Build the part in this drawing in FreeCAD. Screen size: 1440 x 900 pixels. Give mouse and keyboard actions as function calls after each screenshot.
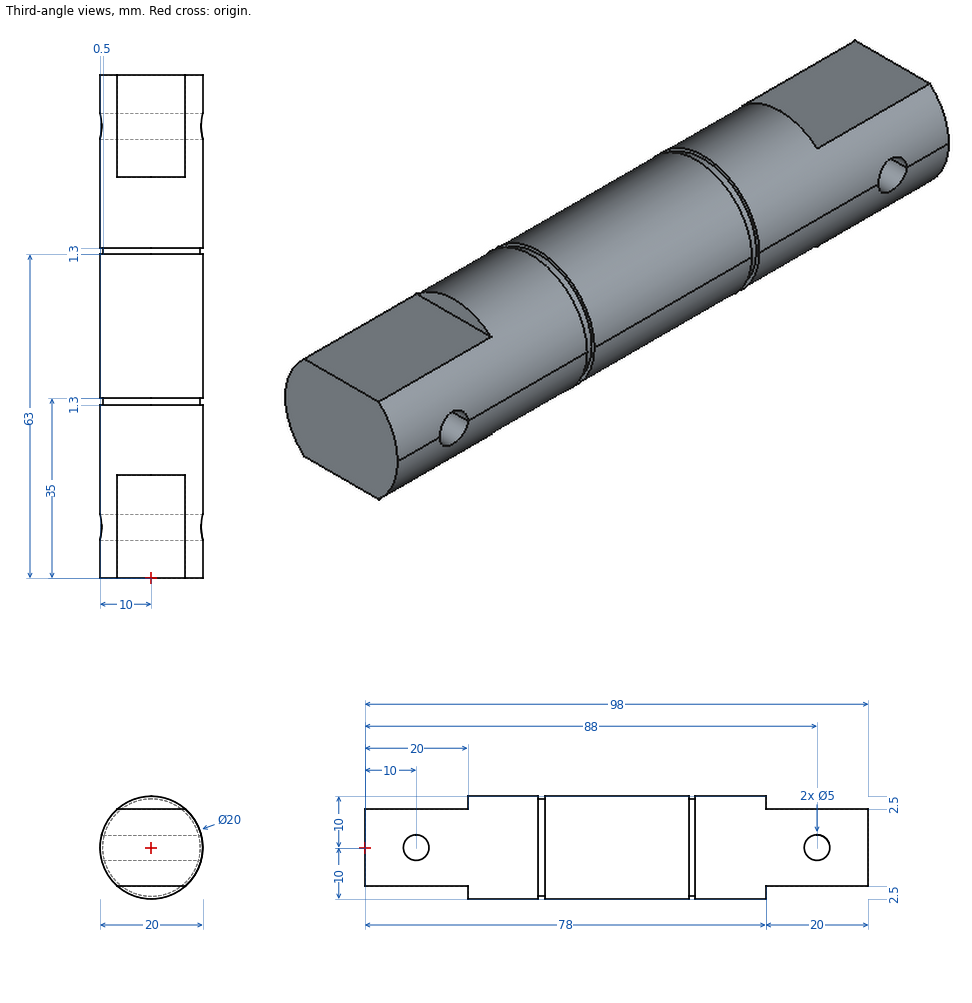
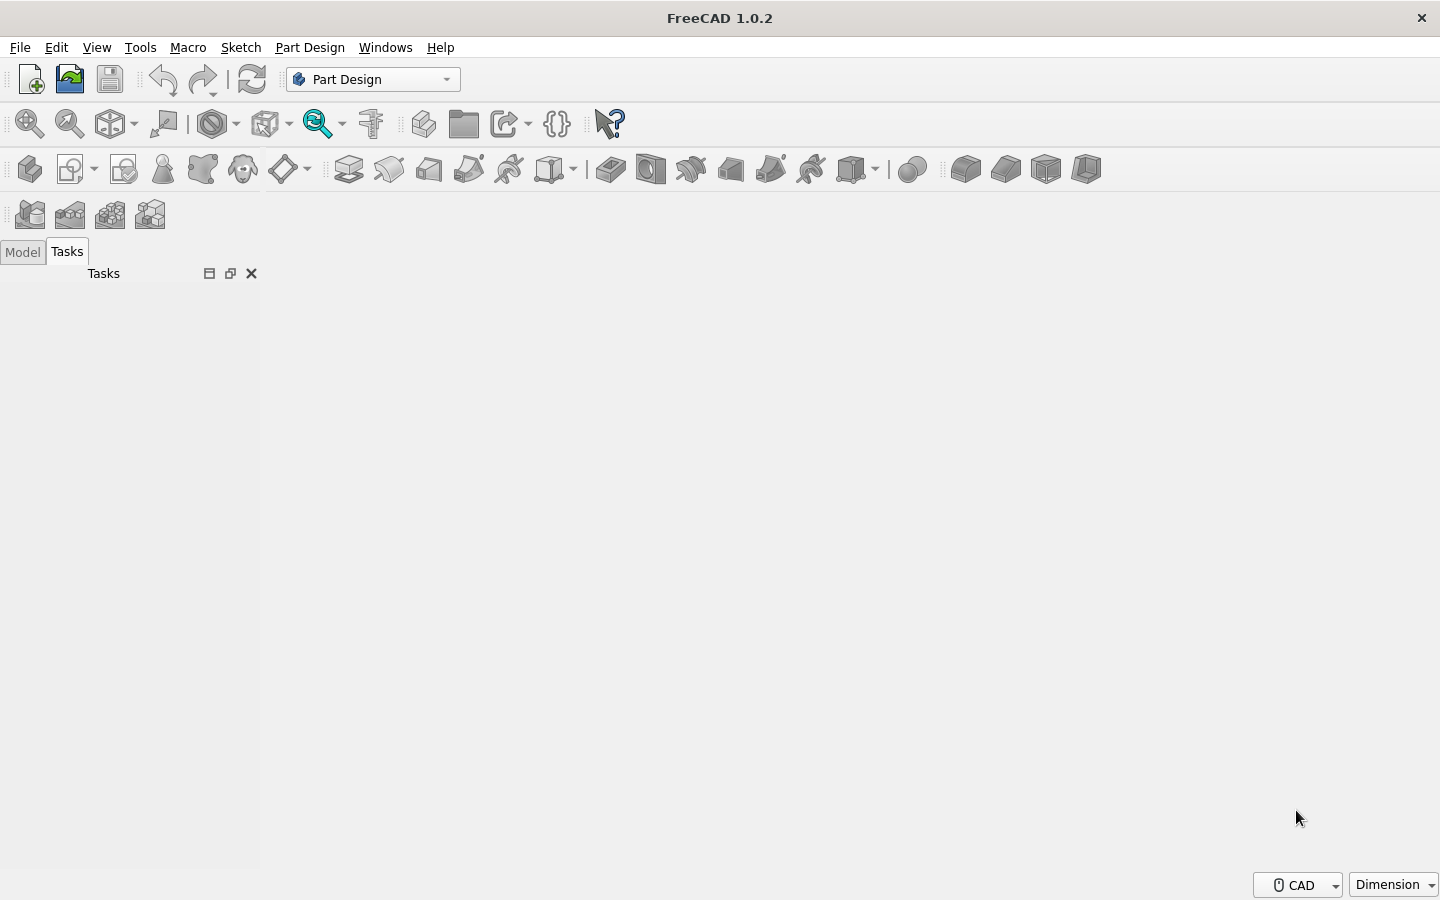
click(30, 80)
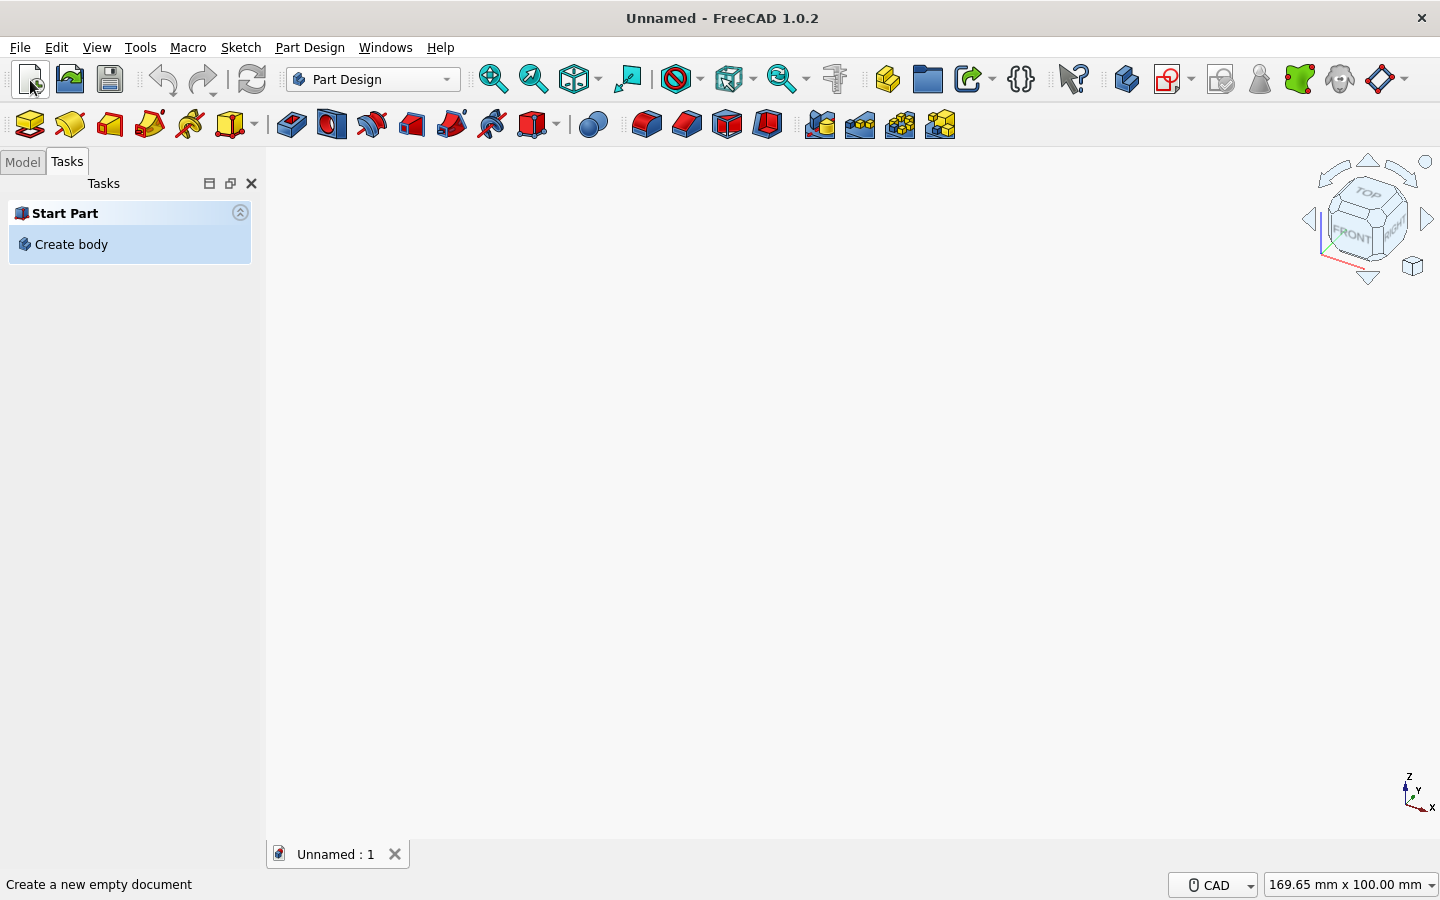
click(1168, 80)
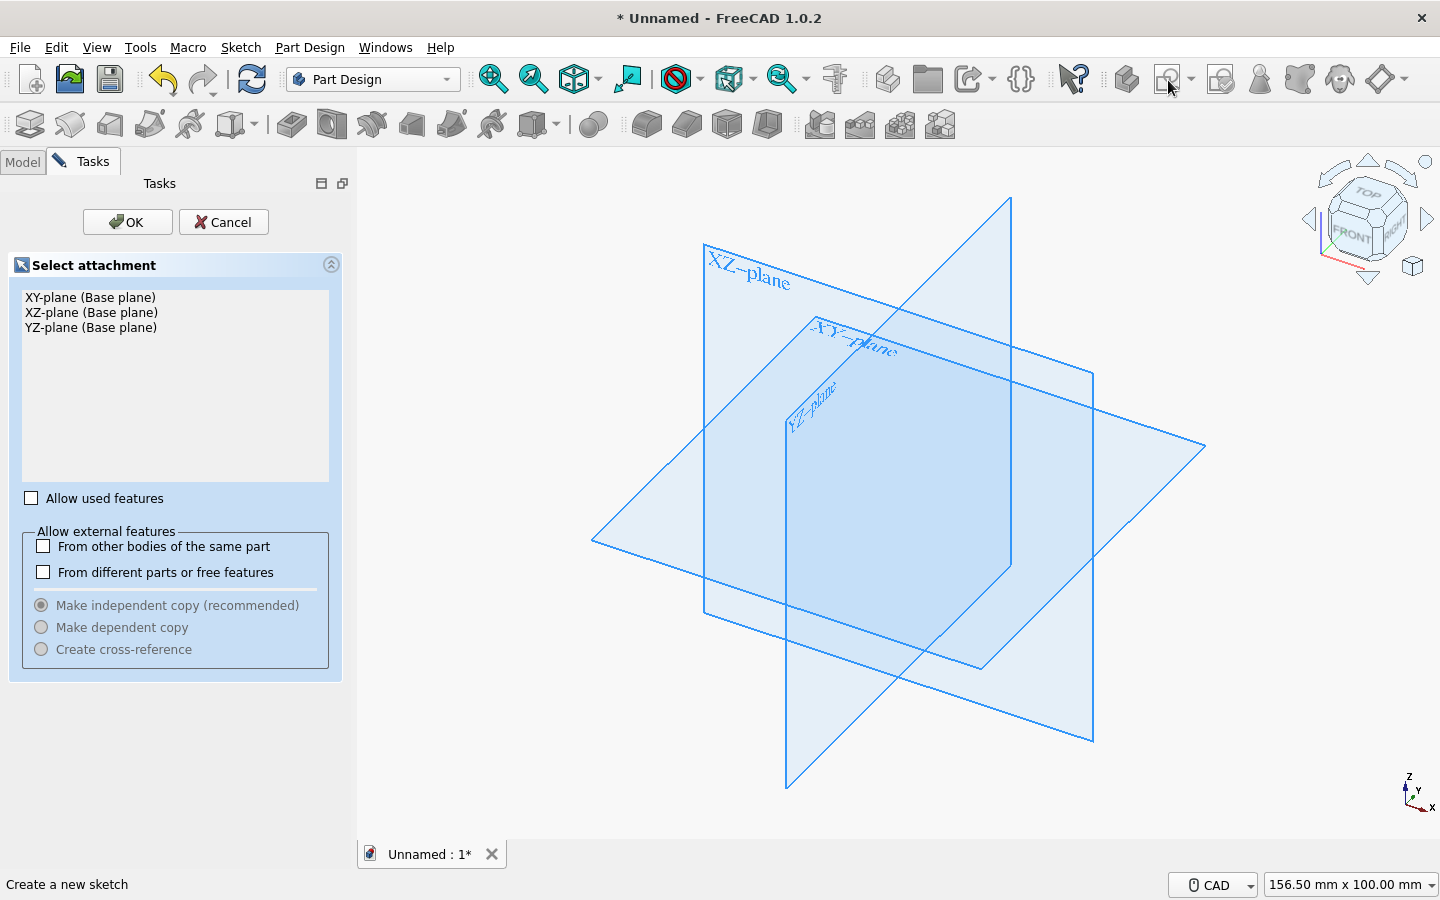
click(82, 312)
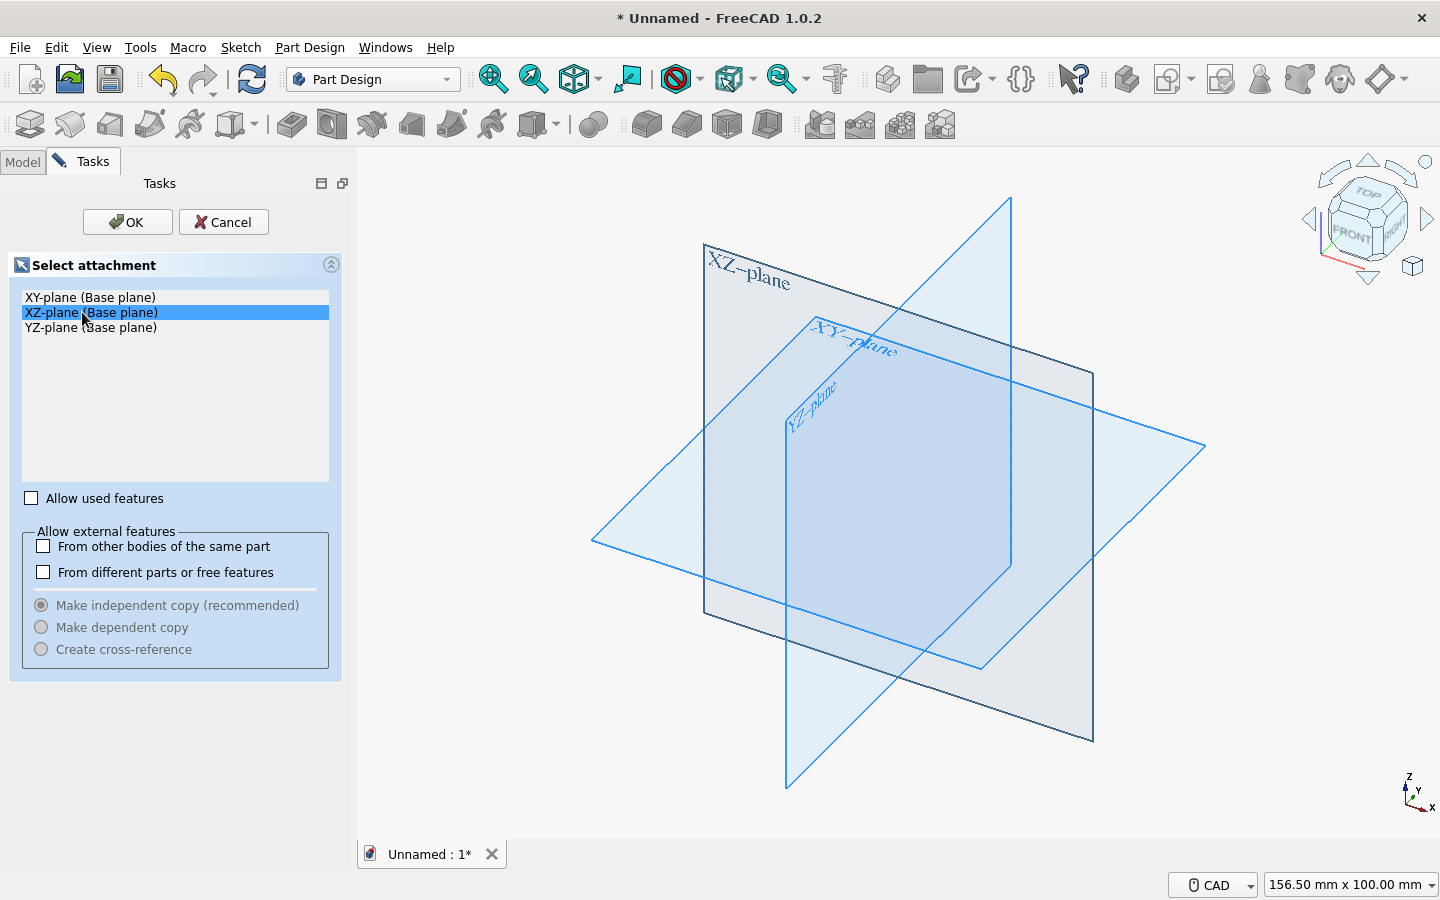
click(128, 222)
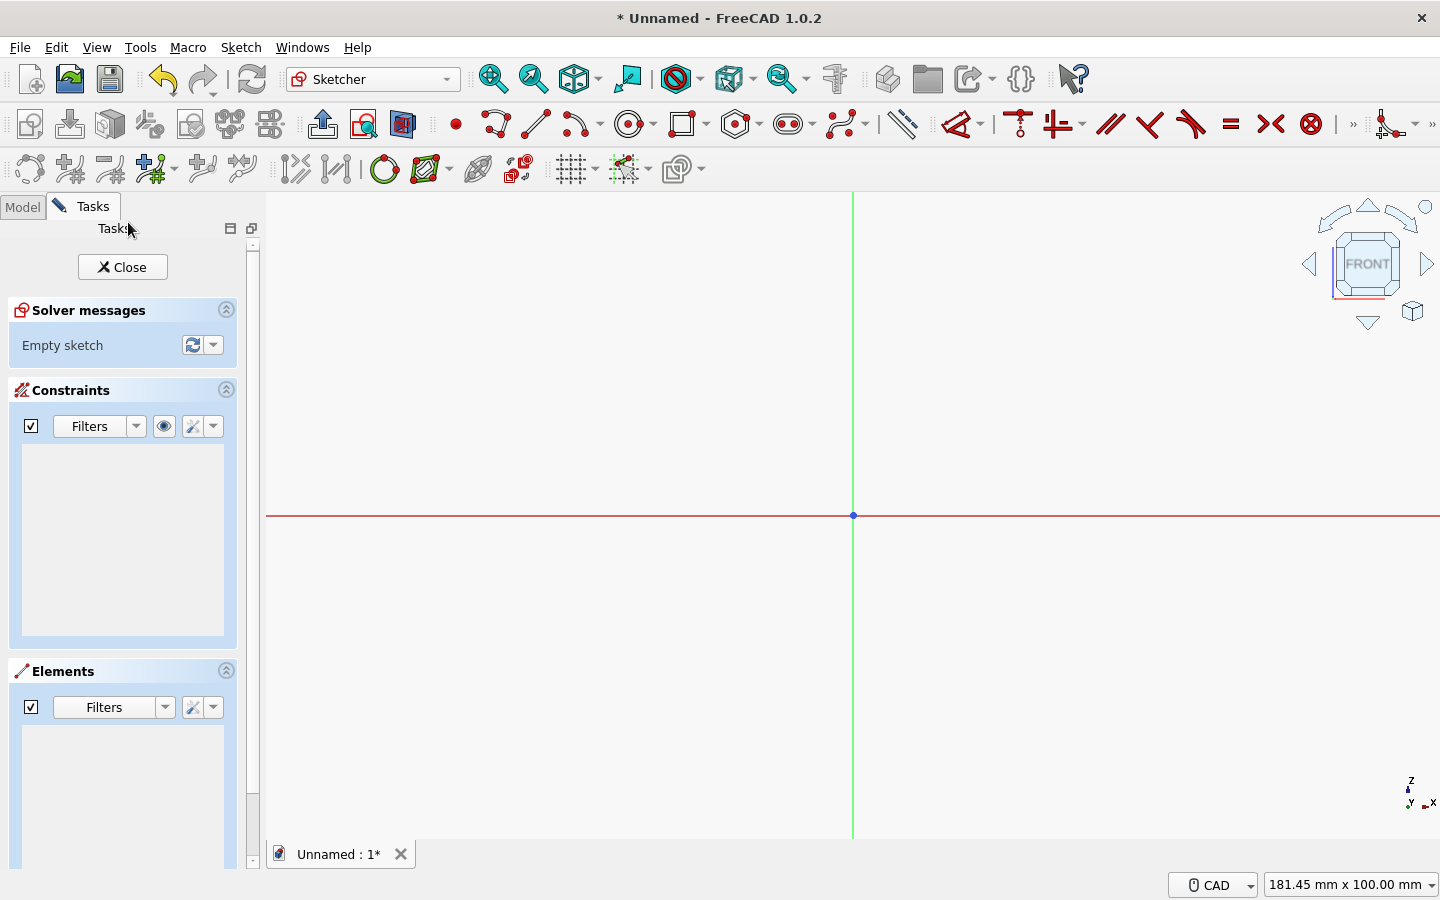
scroll(883, 516, up, 6)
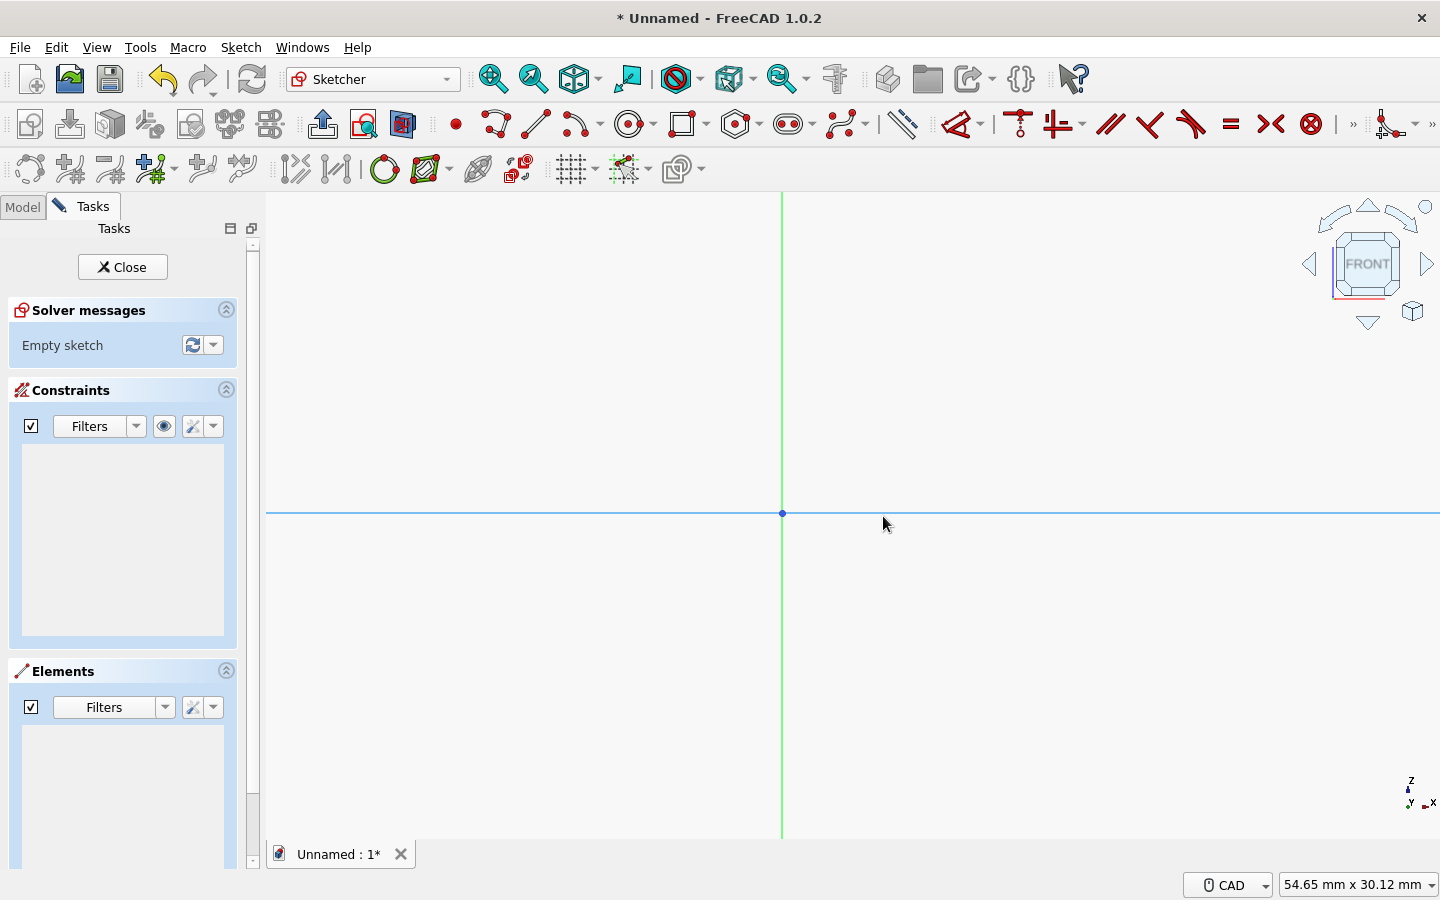
click(630, 124)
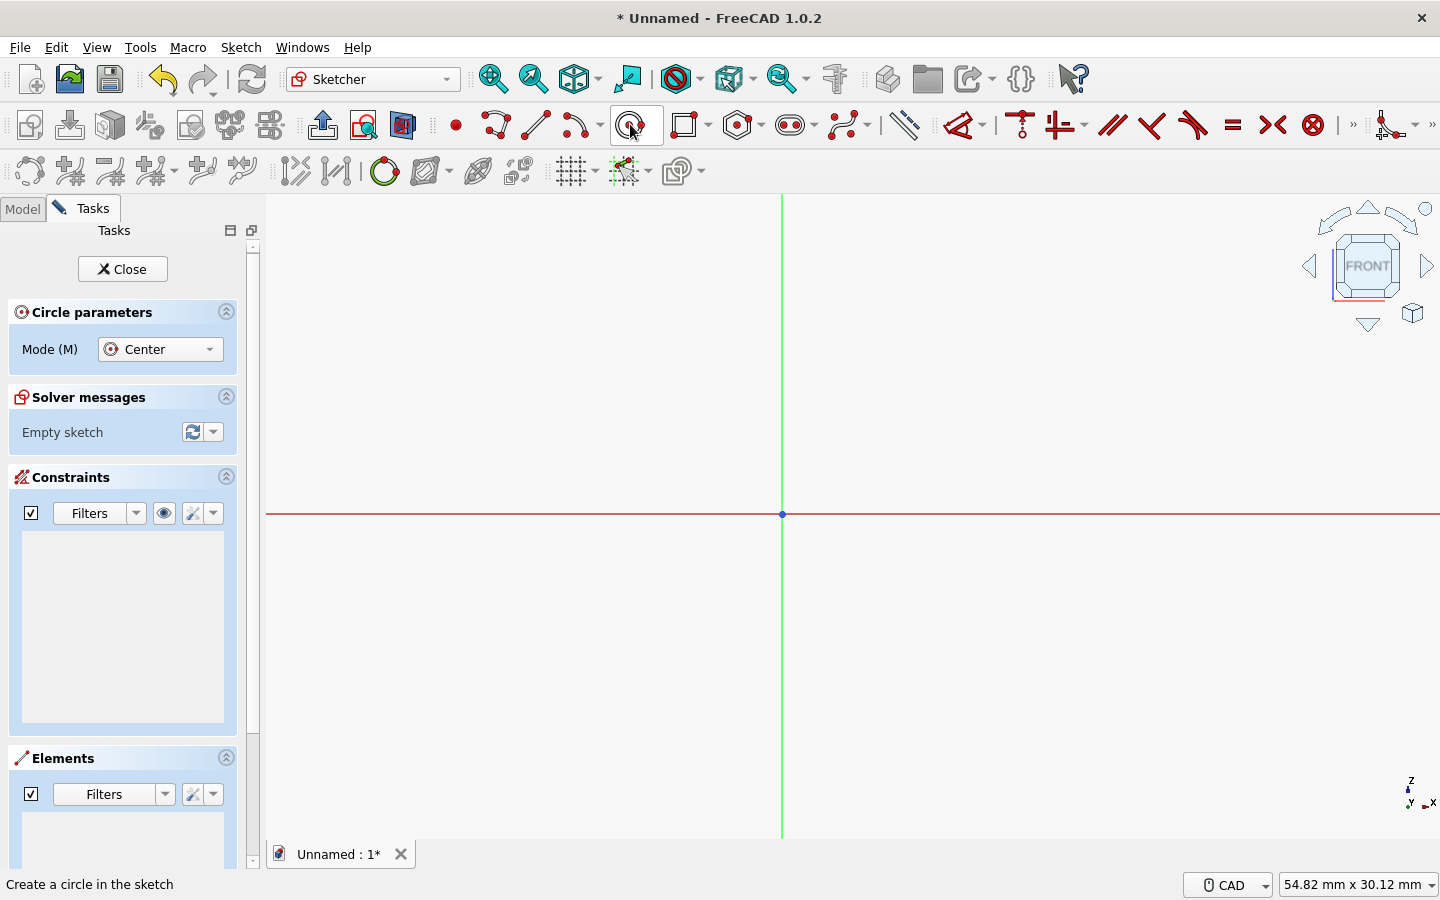
click(782, 514)
move(934, 363)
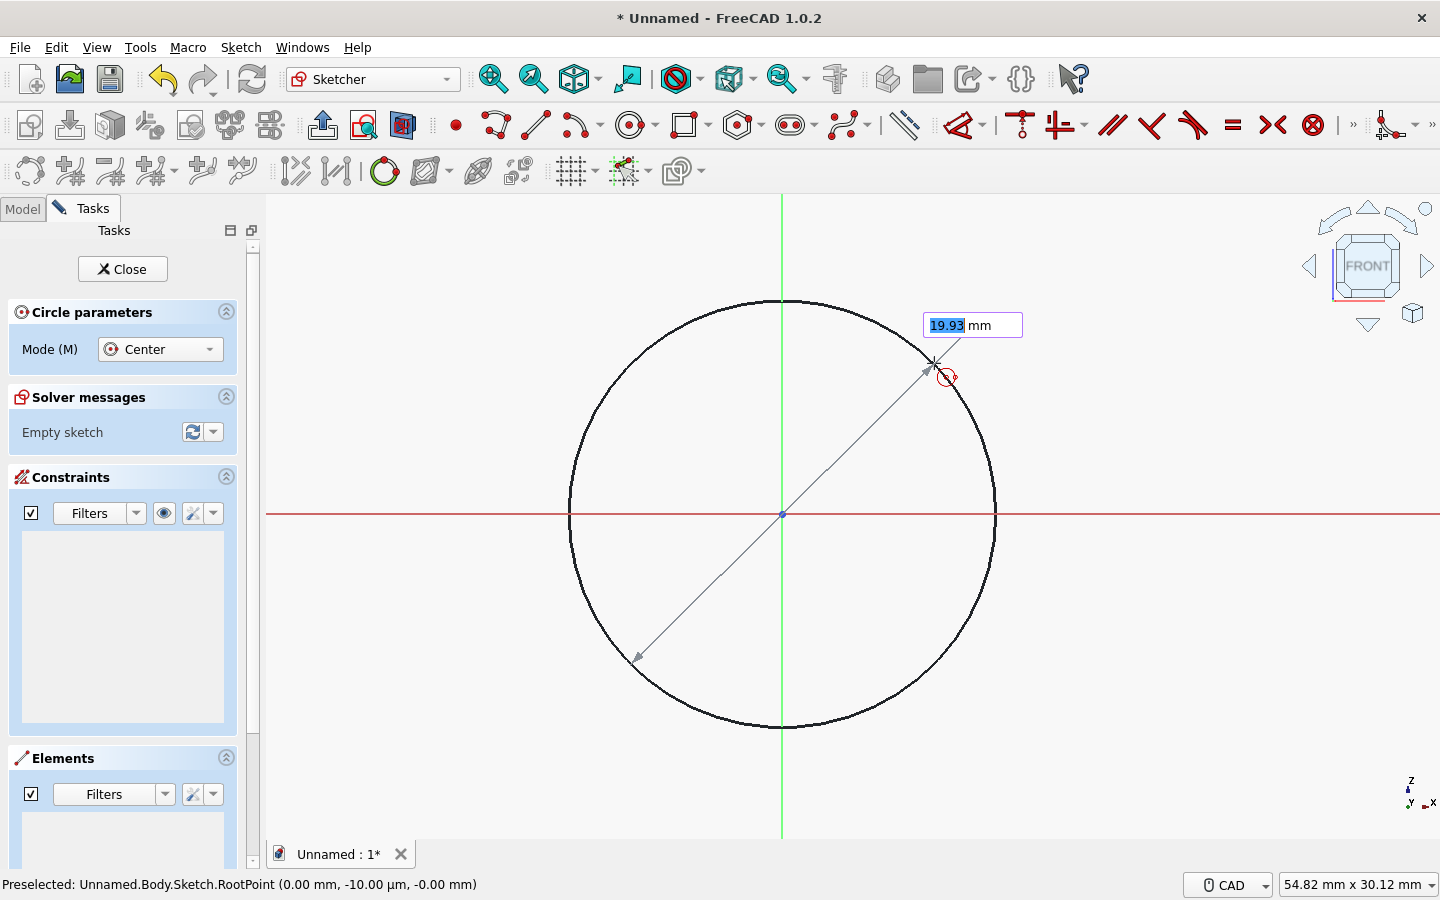
text(20)
key(Return)
key(Escape)